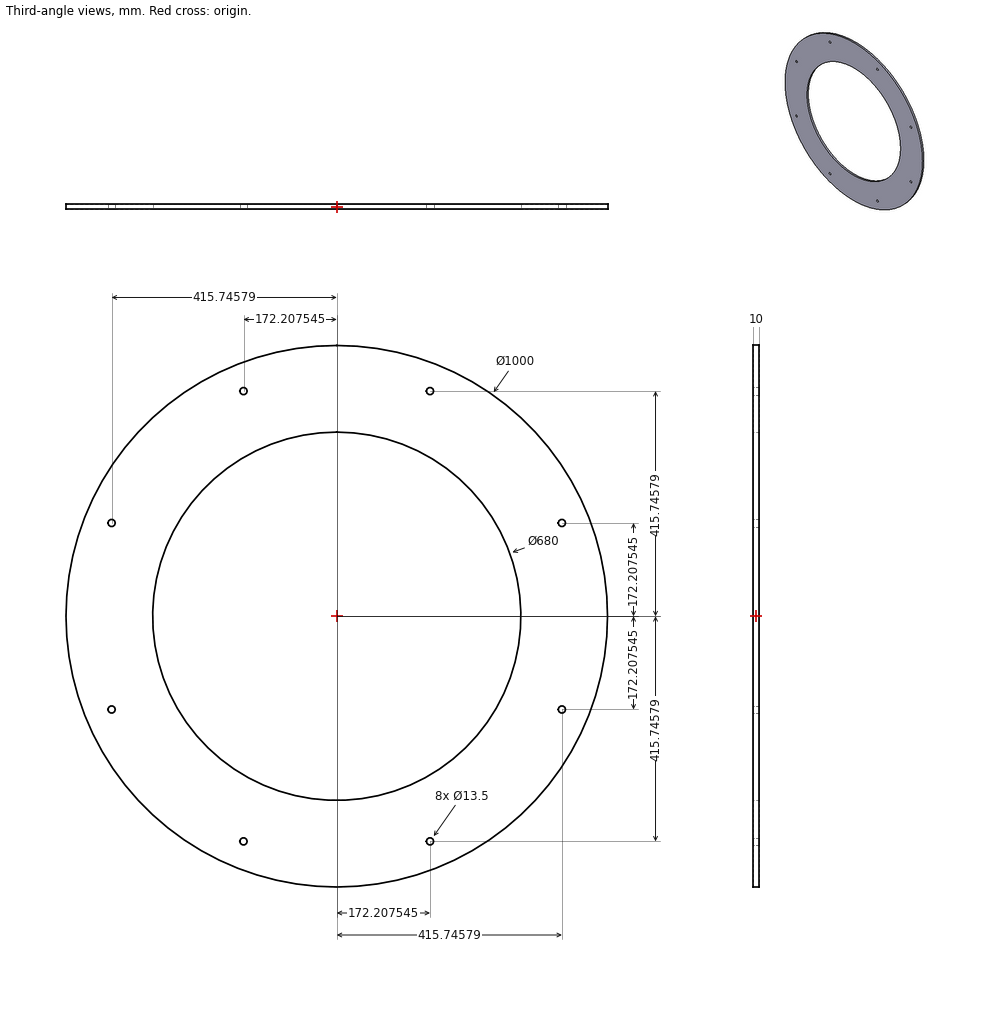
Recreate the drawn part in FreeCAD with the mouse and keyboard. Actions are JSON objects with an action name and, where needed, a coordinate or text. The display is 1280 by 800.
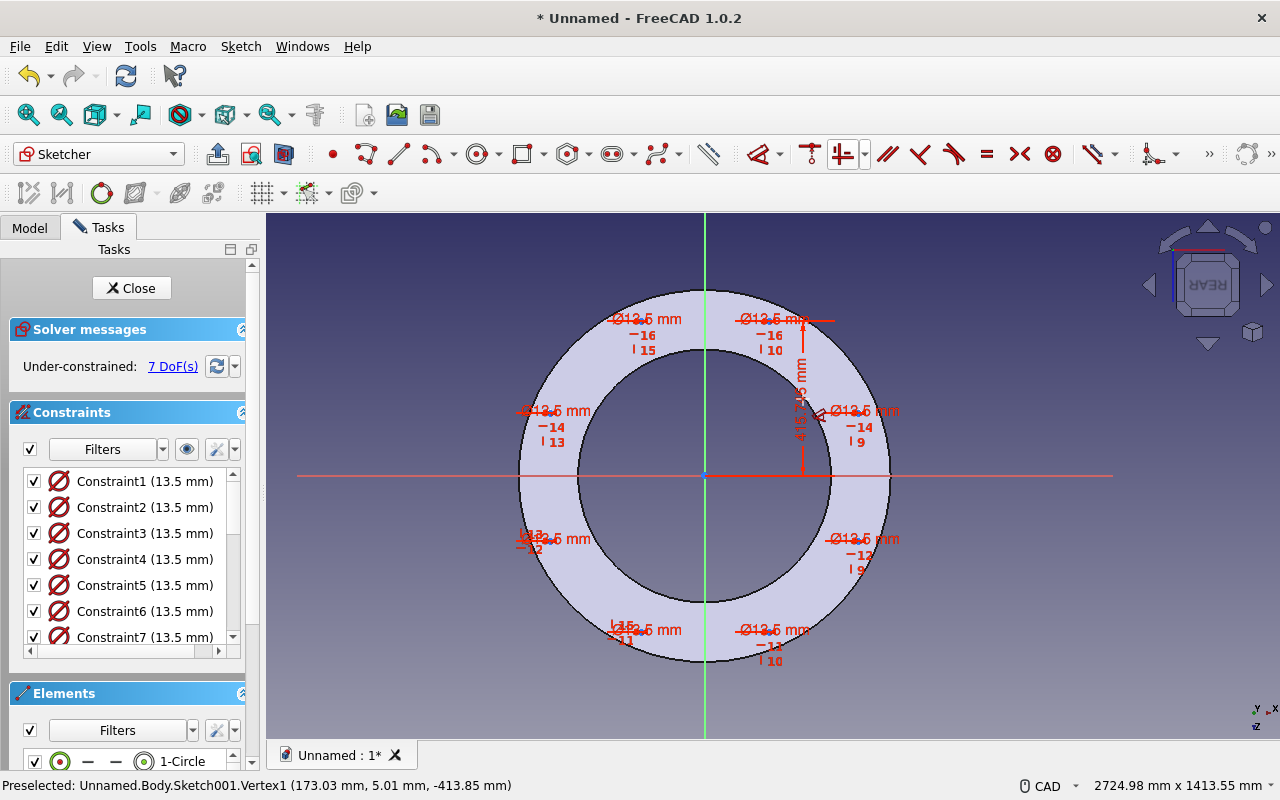
{"action": "left_click", "coordinate": [859, 413]}
{"action": "left_click", "coordinate": [728, 379]}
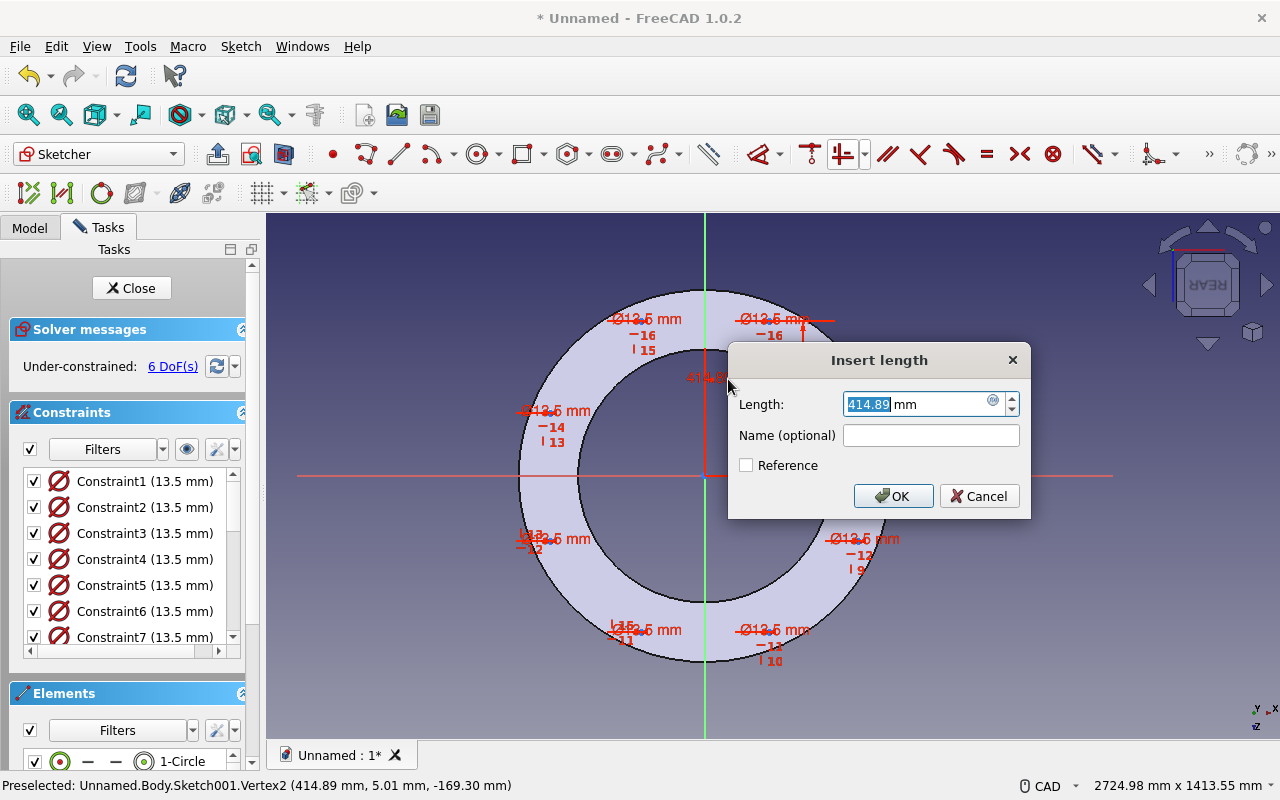
{"action": "type", "text": "415.74579"}
{"action": "key", "text": "Return"}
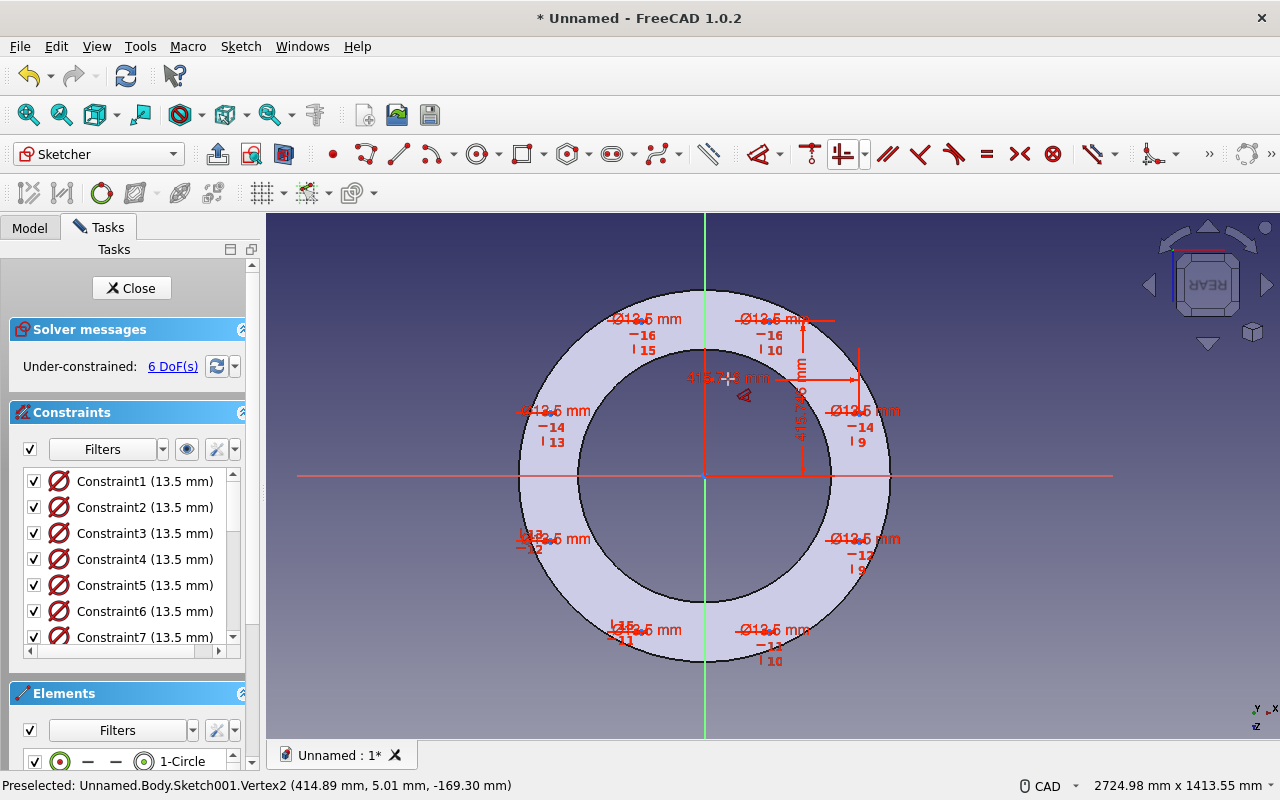
{"action": "left_click", "coordinate": [769, 632]}
{"action": "left_click", "coordinate": [803, 554]}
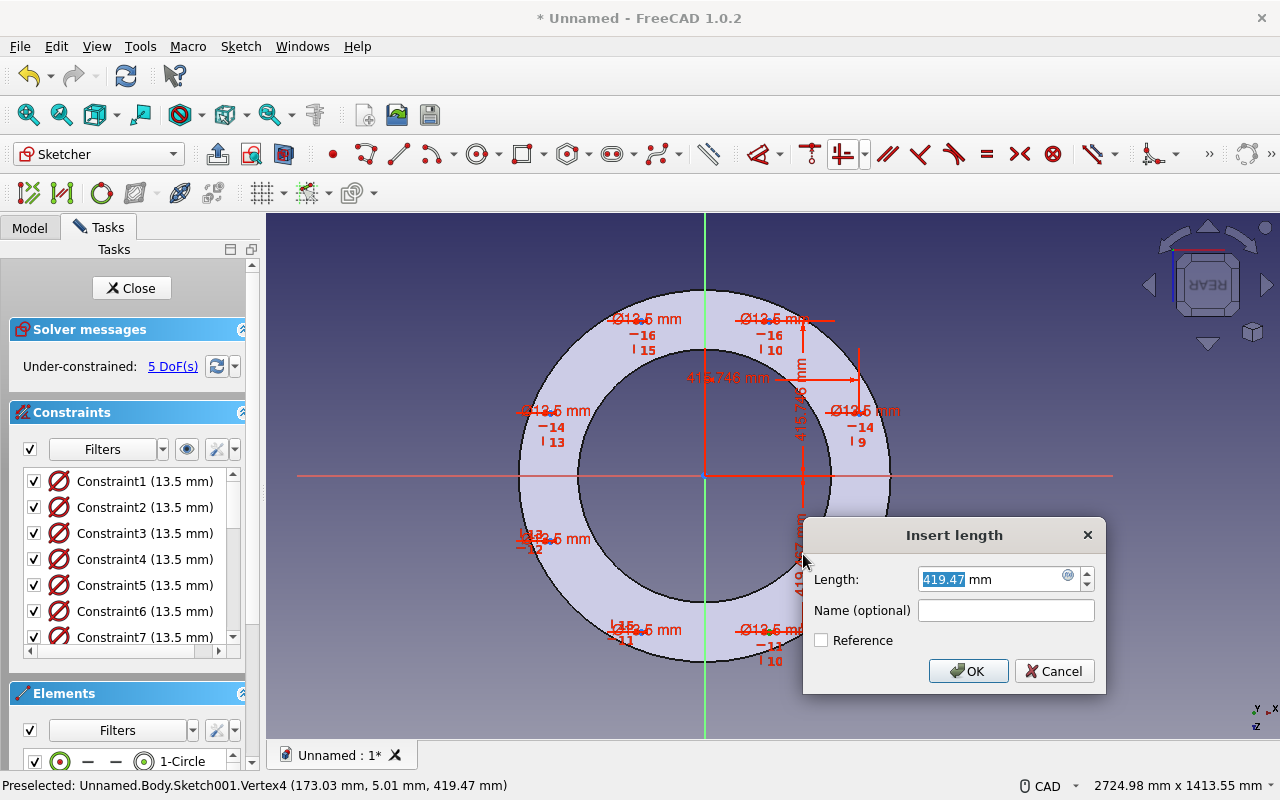
{"action": "type", "text": "415.74579"}
{"action": "key", "text": "Return"}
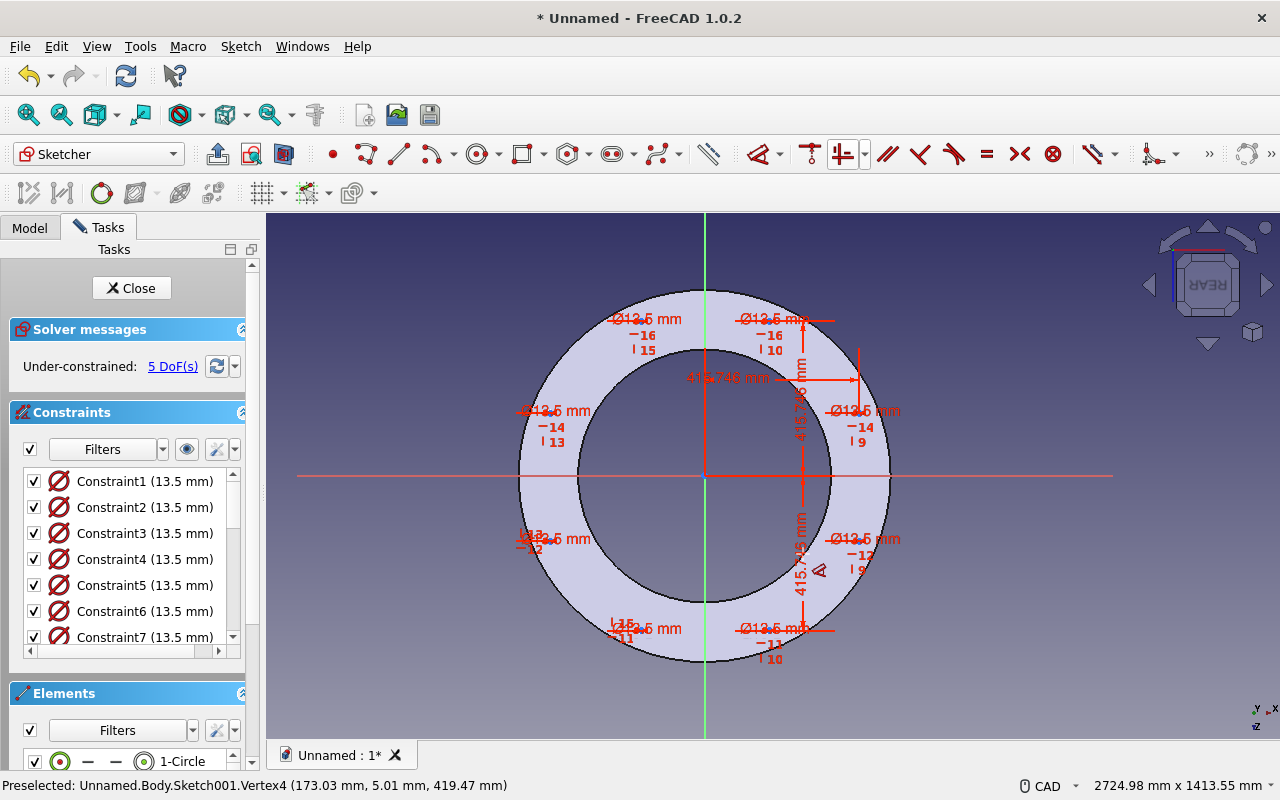
{"action": "left_click", "coordinate": [550, 541]}
{"action": "left_click", "coordinate": [627, 575]}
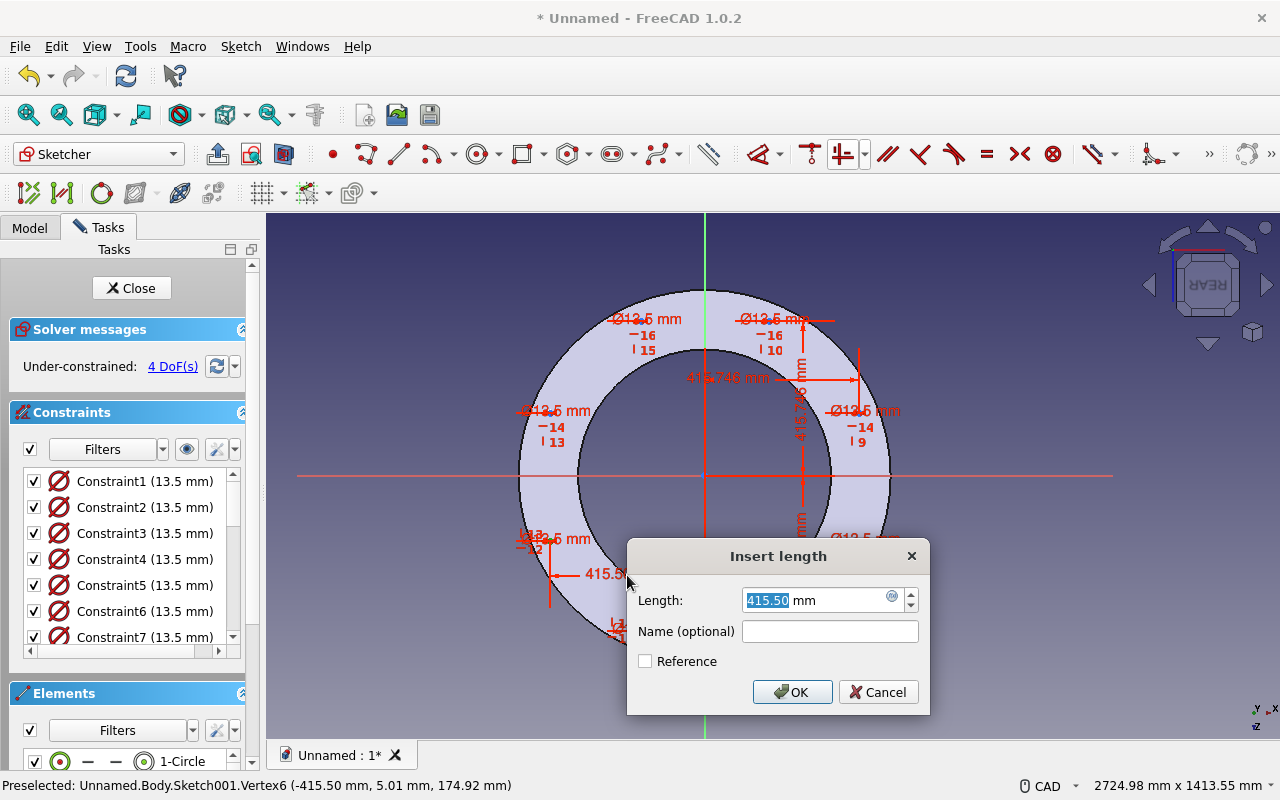
{"action": "type", "text": "415.74579"}
{"action": "key", "text": "Return"}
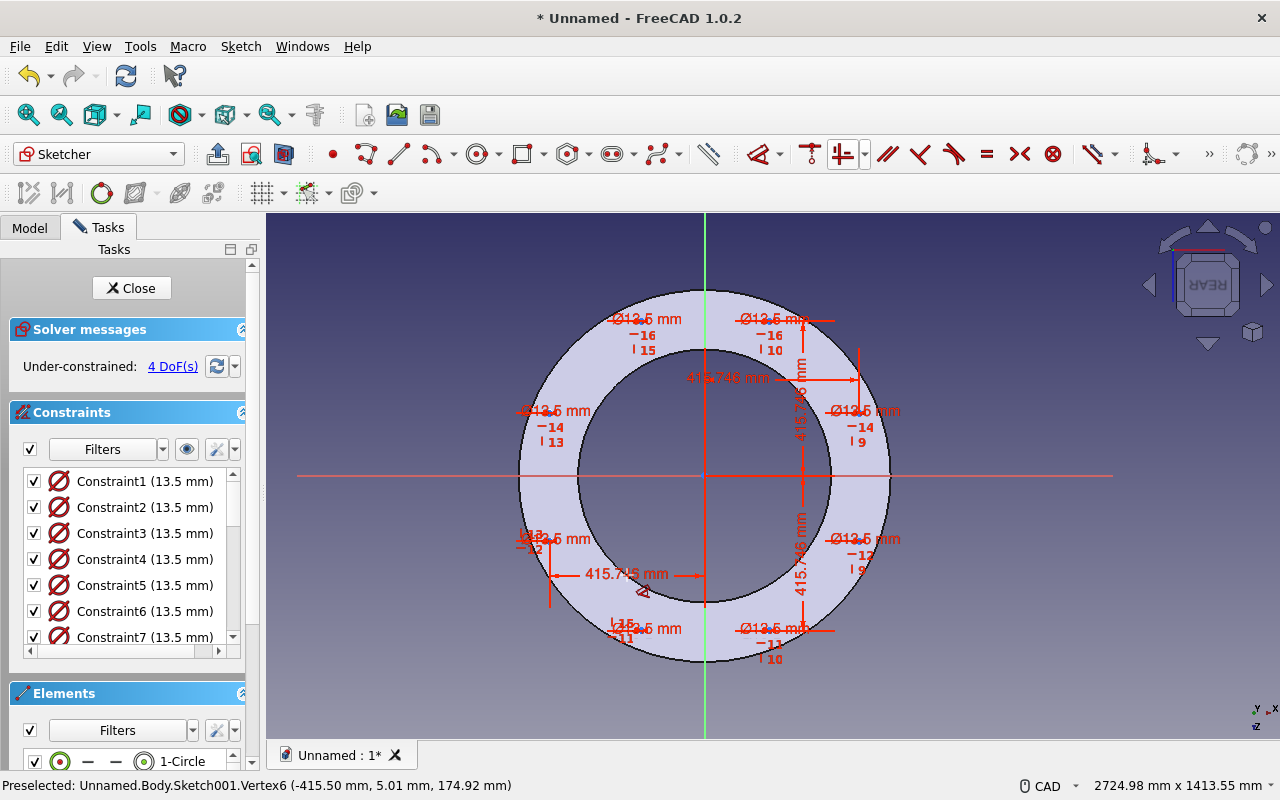
{"action": "left_click", "coordinate": [769, 321]}
{"action": "left_click", "coordinate": [737, 287]}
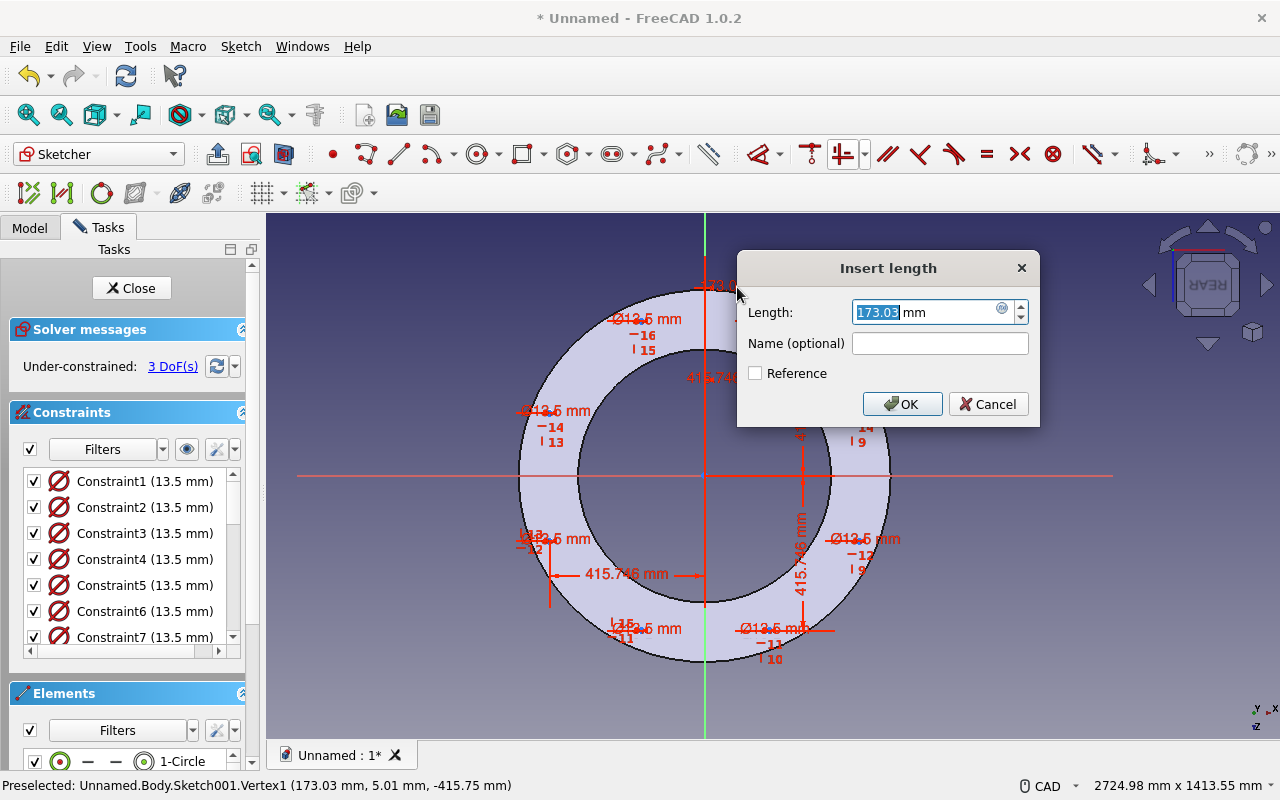
{"action": "type", "text": "172.207545"}
{"action": "key", "text": "Return"}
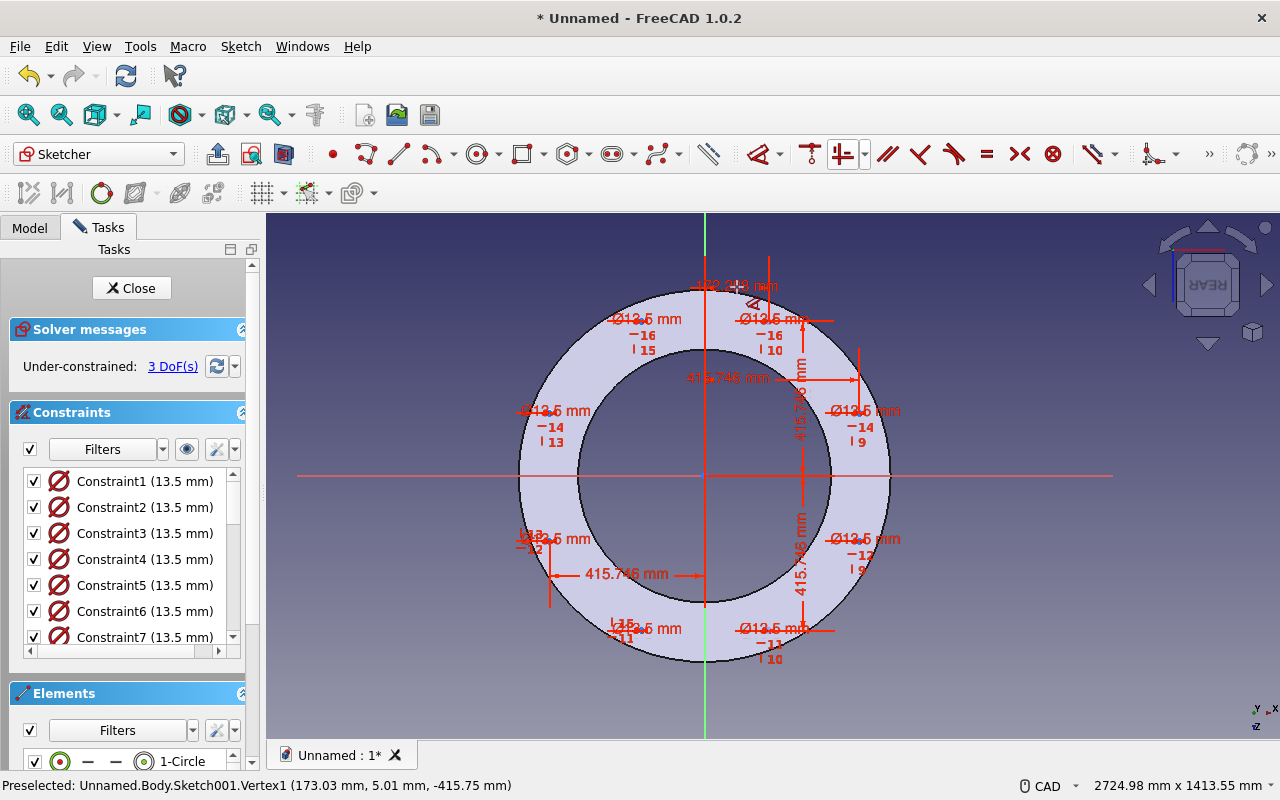
{"action": "left_click", "coordinate": [859, 413]}
{"action": "left_click", "coordinate": [893, 445]}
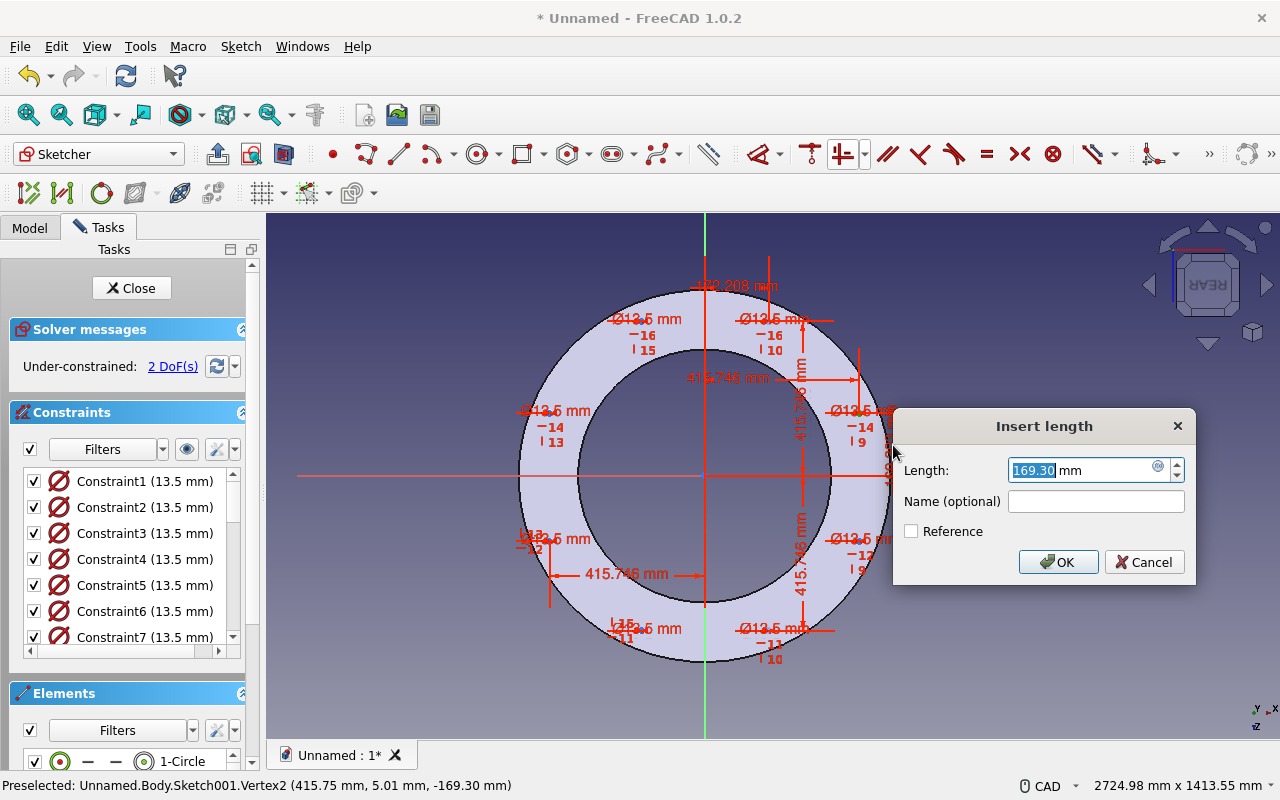
{"action": "type", "text": "172.207545"}
{"action": "key", "text": "Return"}